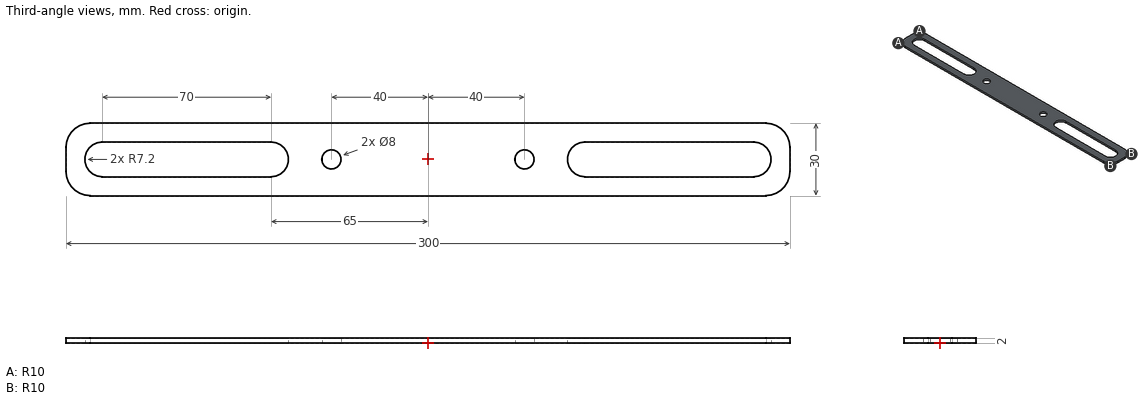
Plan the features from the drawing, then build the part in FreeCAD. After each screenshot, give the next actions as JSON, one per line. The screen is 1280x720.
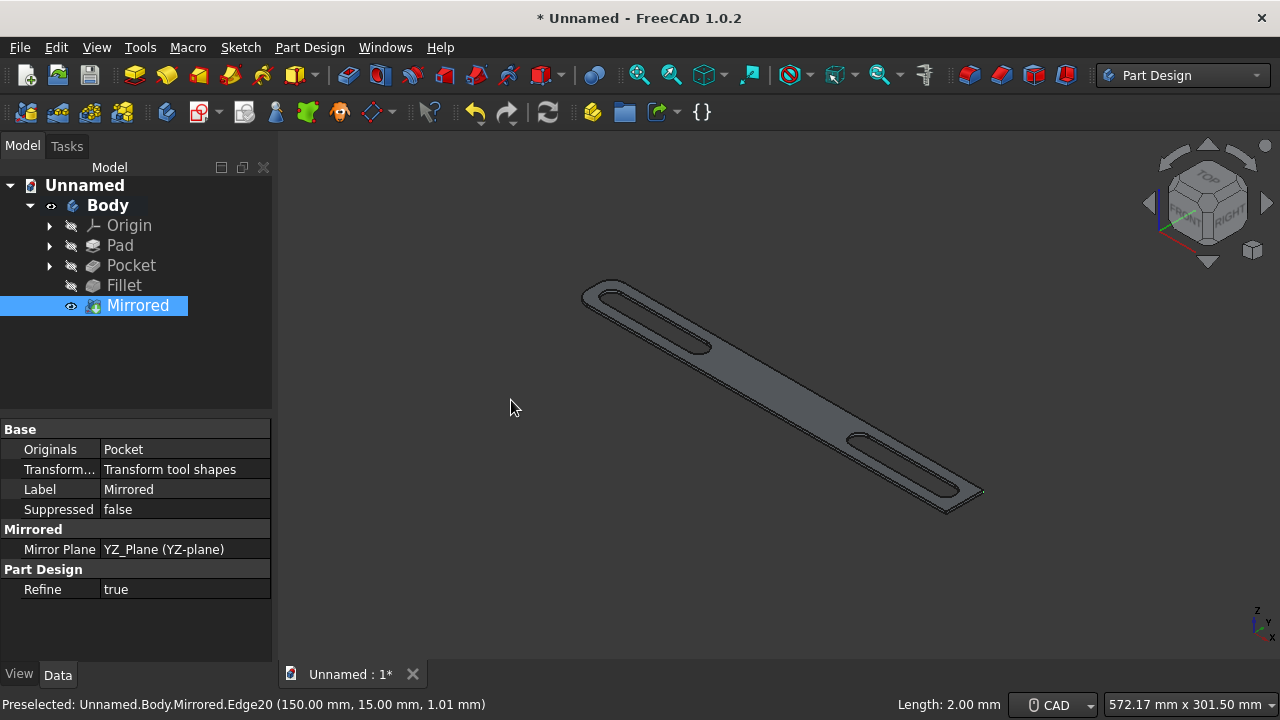
{"action": "scroll", "coordinate": [946, 512], "scroll_direction": "up", "scroll_amount": 13}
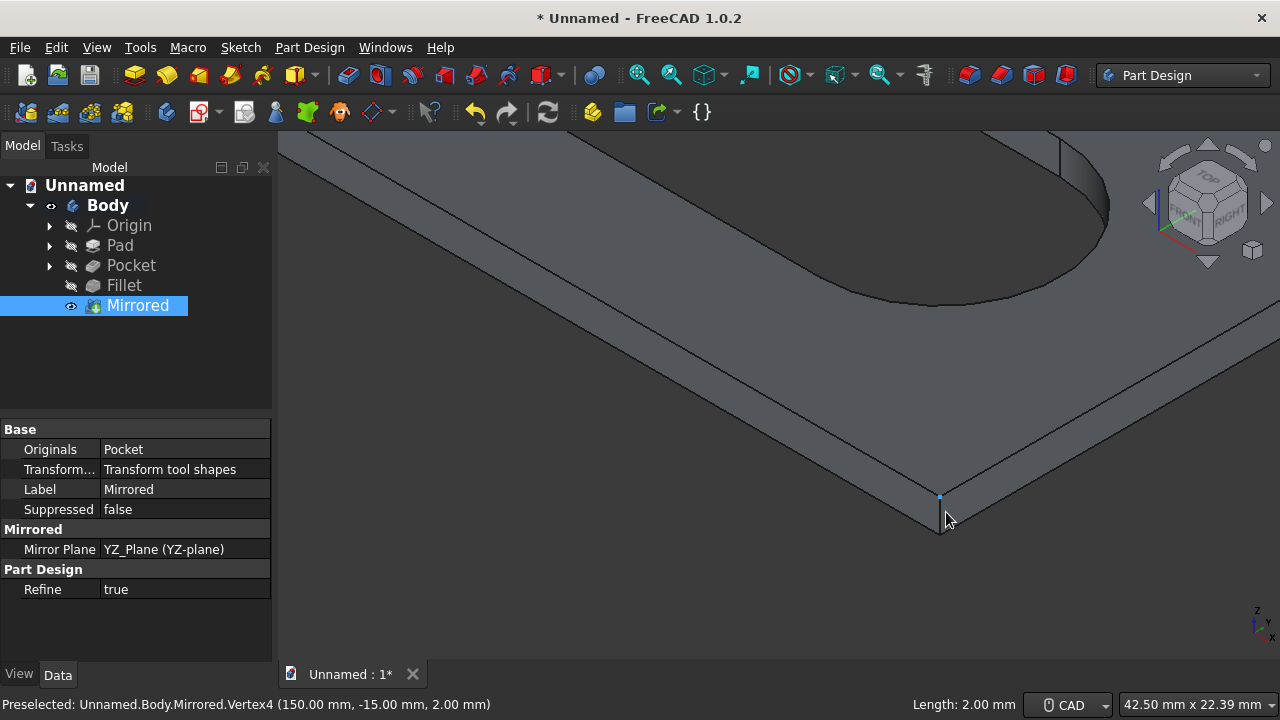
{"action": "left_click", "coordinate": [940, 515], "text": "ctrl"}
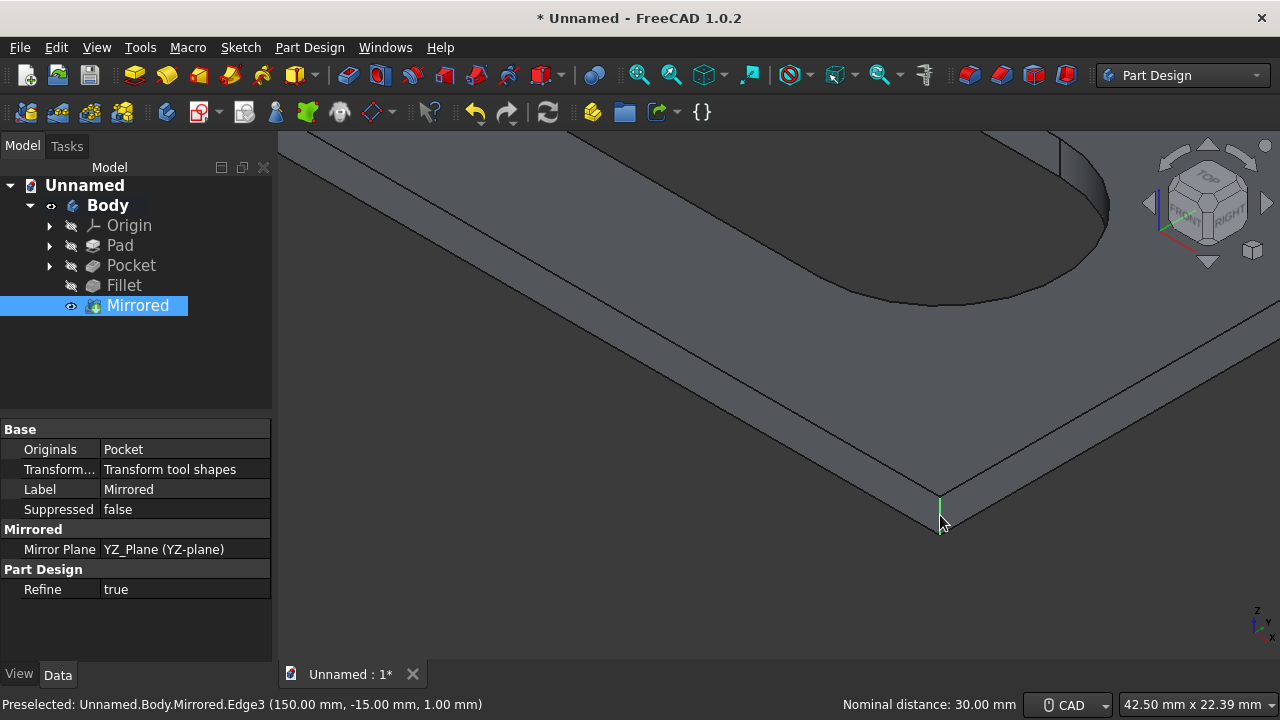
{"action": "left_click", "coordinate": [970, 76]}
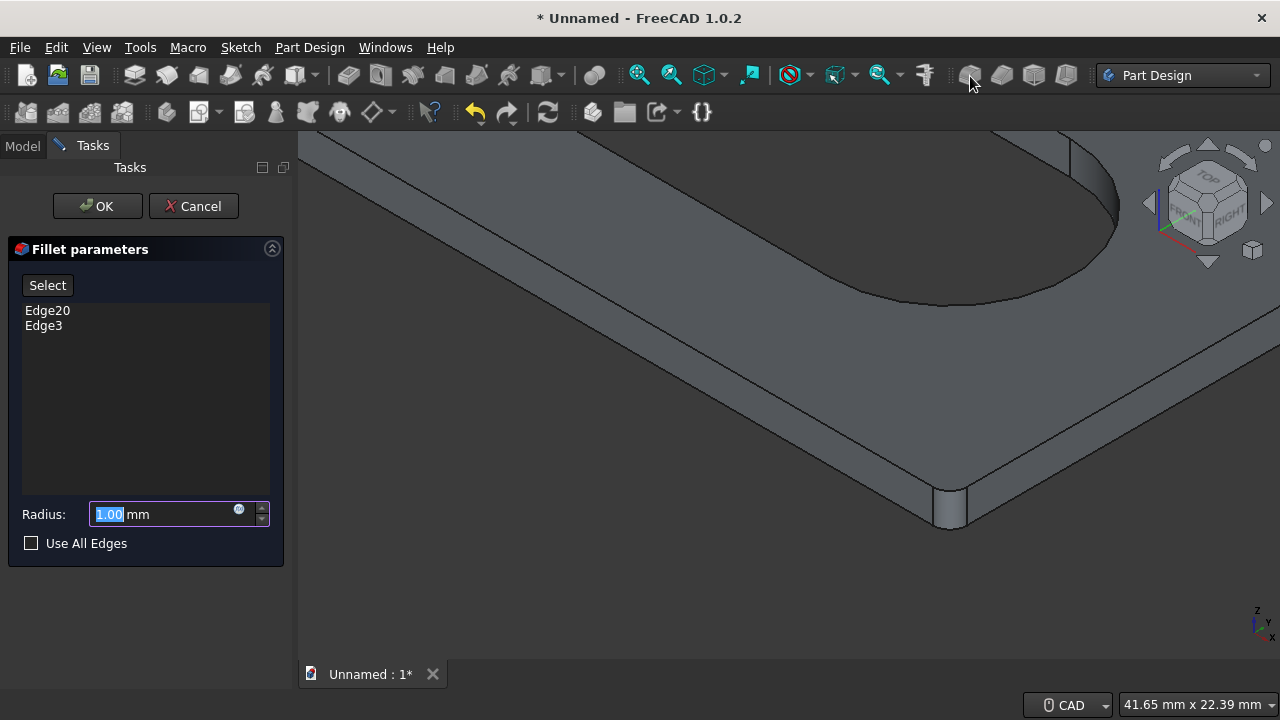
{"action": "type", "text": "10"}
{"action": "key", "text": "Tab"}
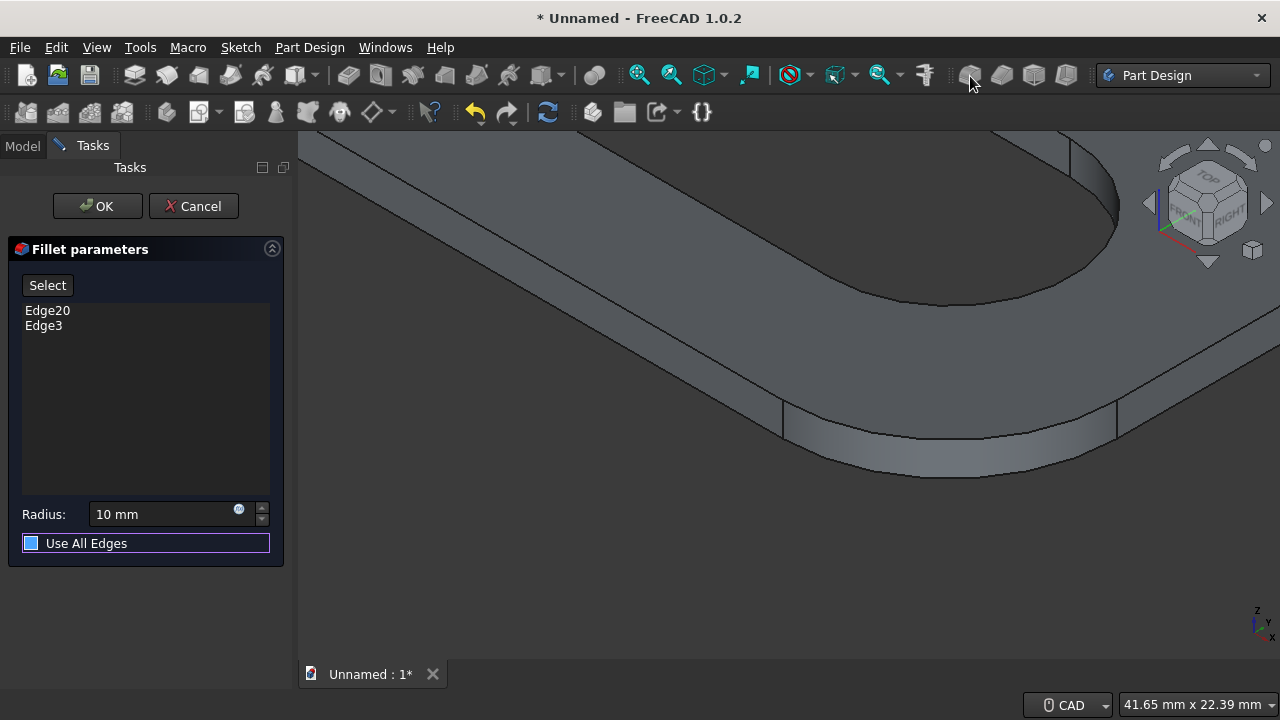
{"action": "left_click", "coordinate": [98, 206]}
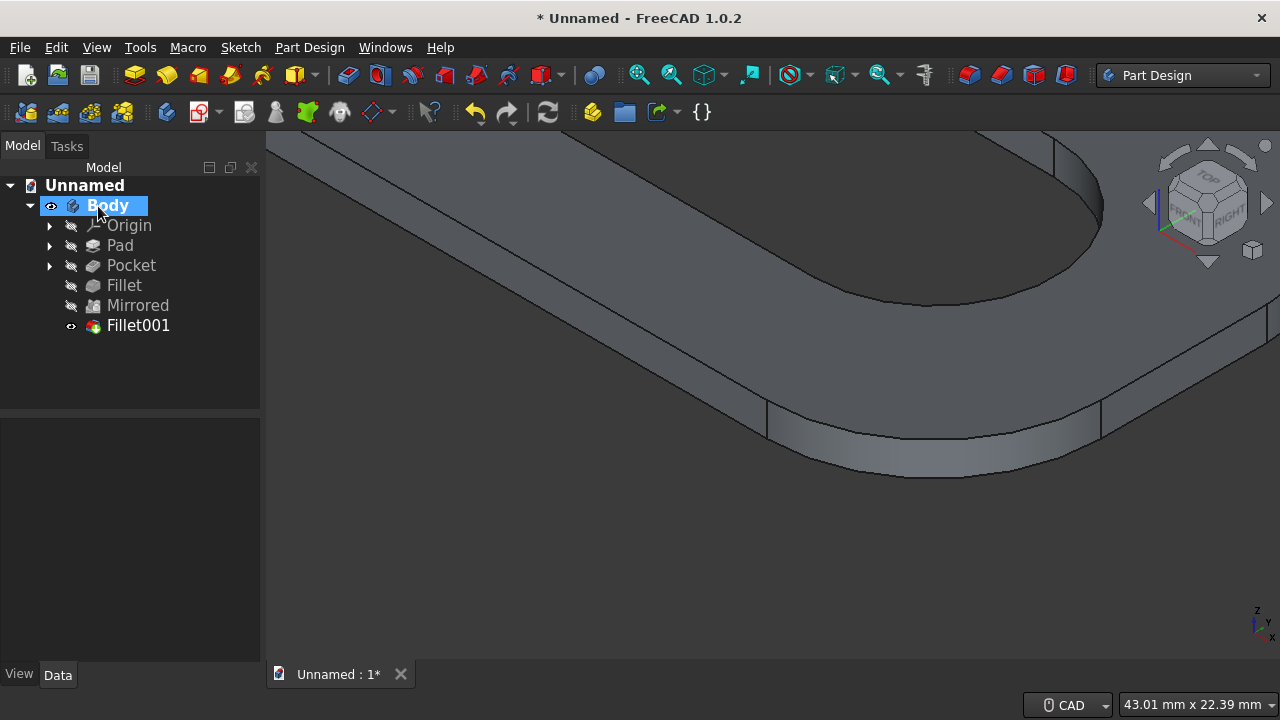
{"action": "key", "text": "v f"}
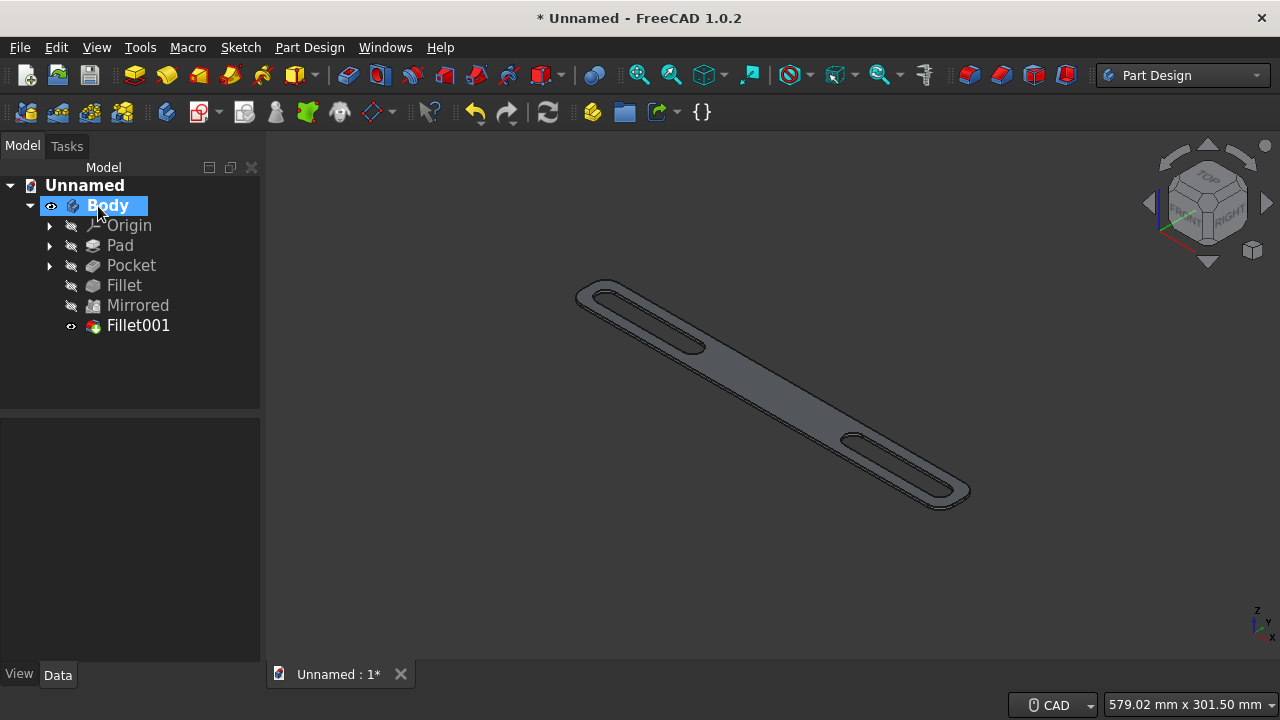
{"action": "left_click", "coordinate": [200, 112]}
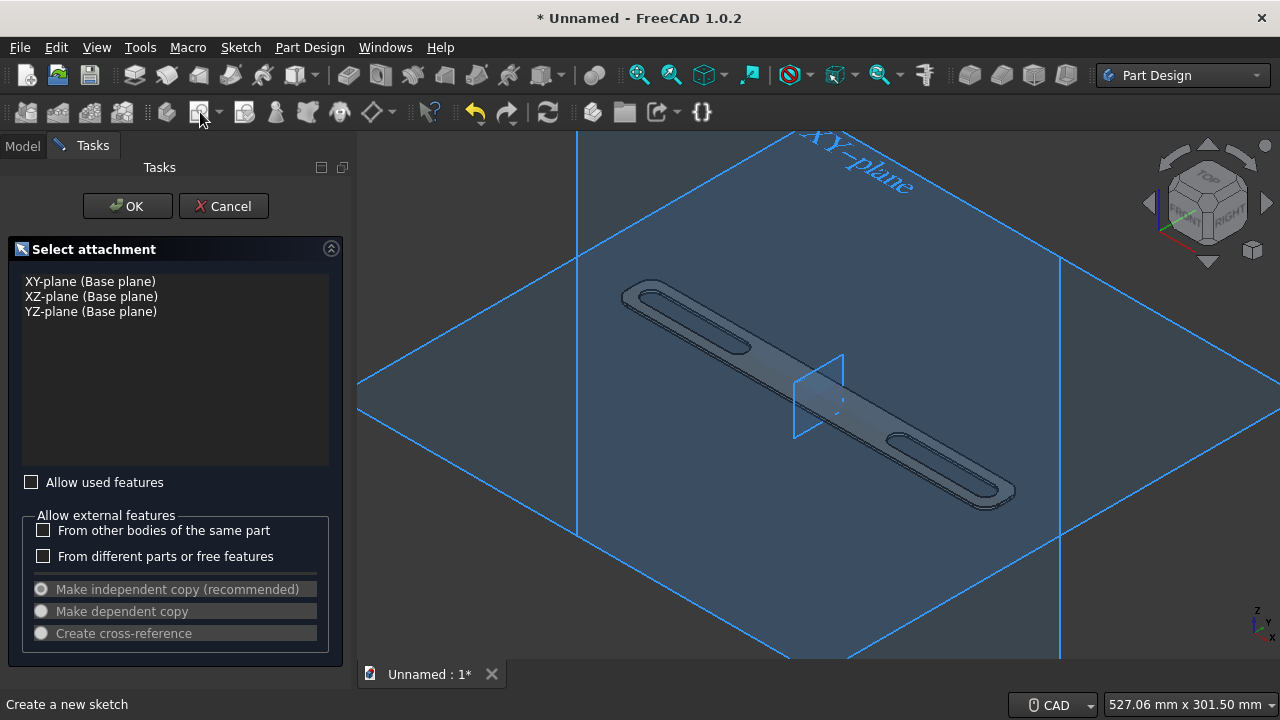
{"action": "left_click", "coordinate": [82, 282]}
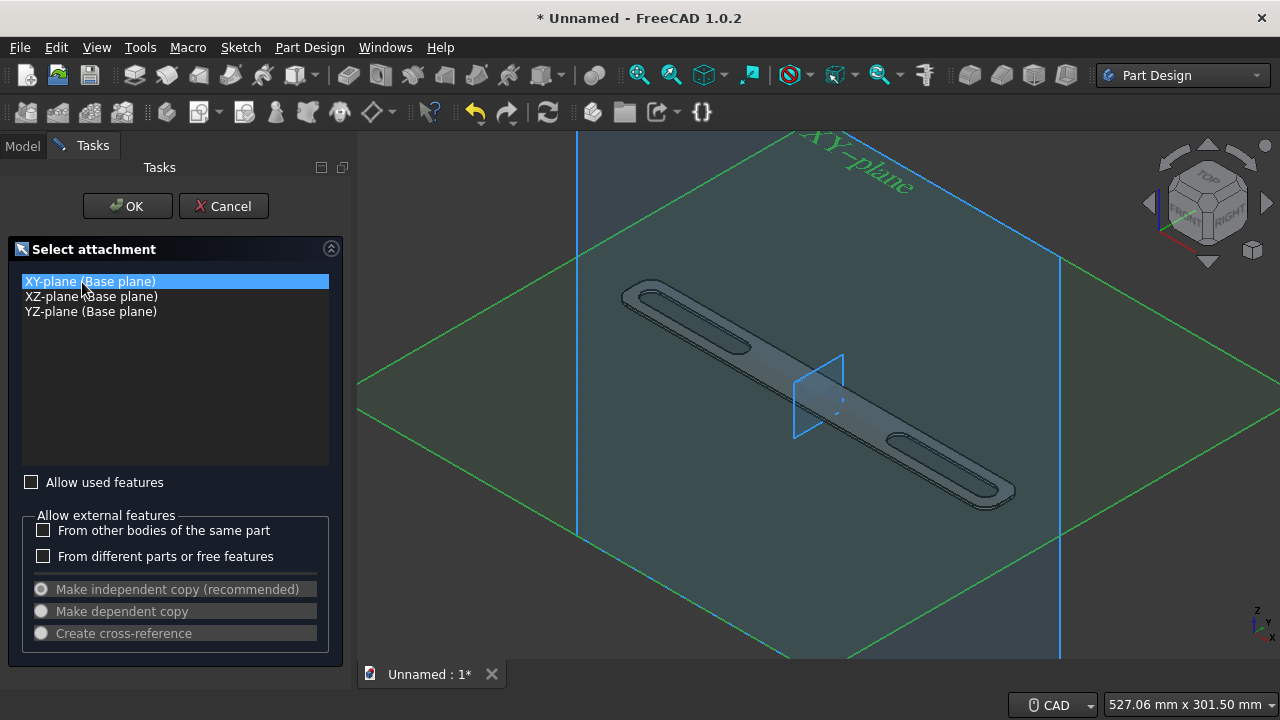
{"action": "left_click", "coordinate": [128, 206]}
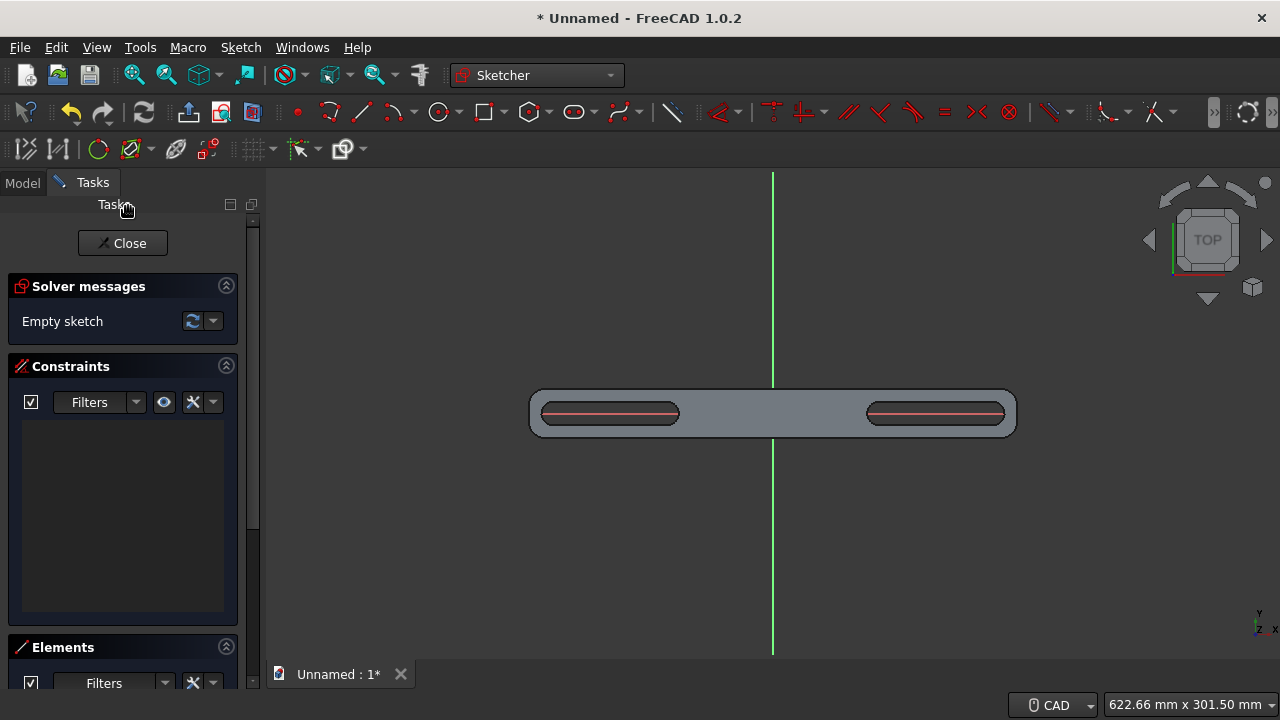
{"action": "left_click", "coordinate": [254, 112]}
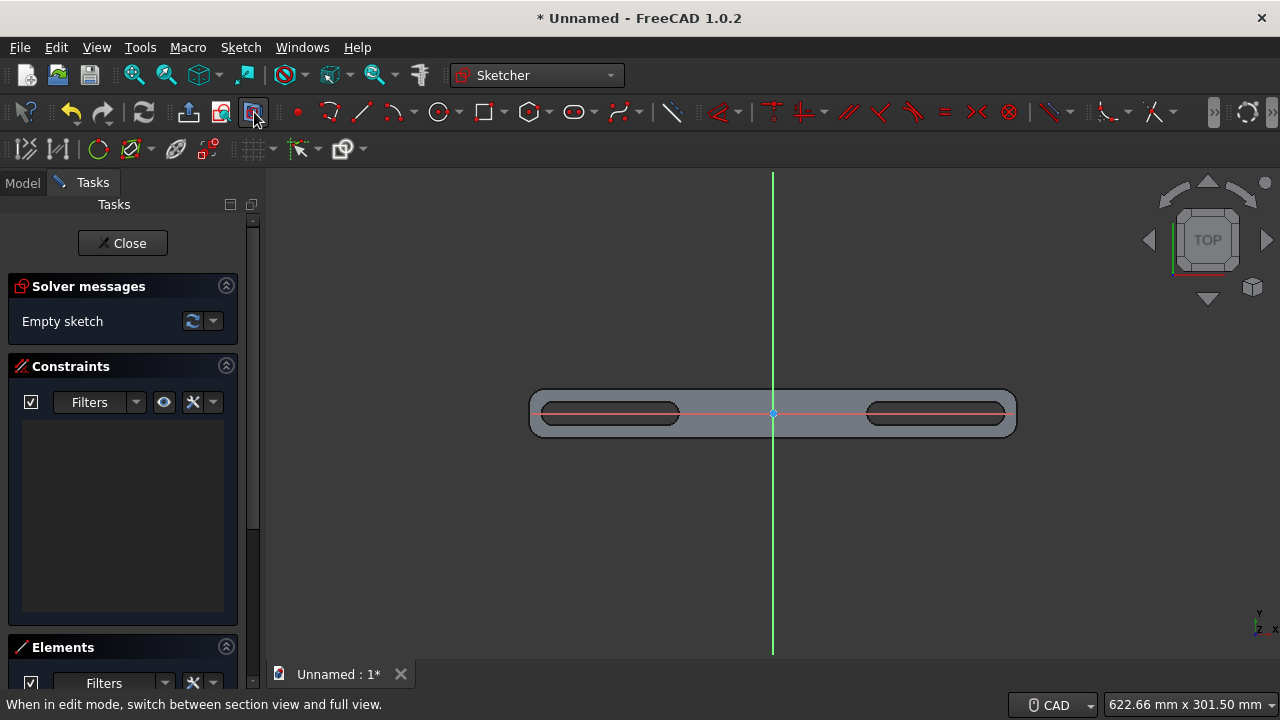
{"action": "scroll", "coordinate": [795, 414], "scroll_direction": "up", "scroll_amount": 7}